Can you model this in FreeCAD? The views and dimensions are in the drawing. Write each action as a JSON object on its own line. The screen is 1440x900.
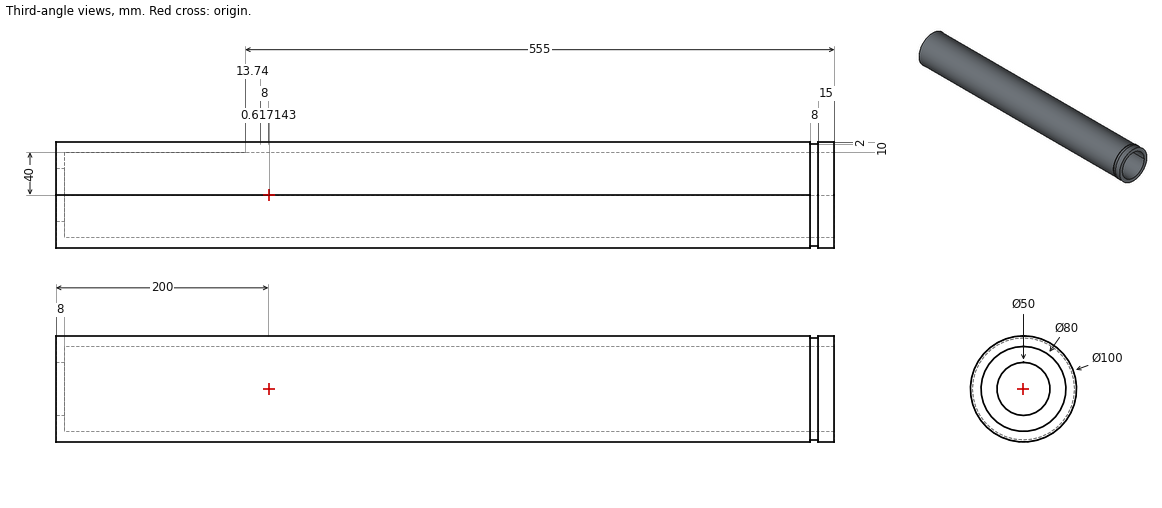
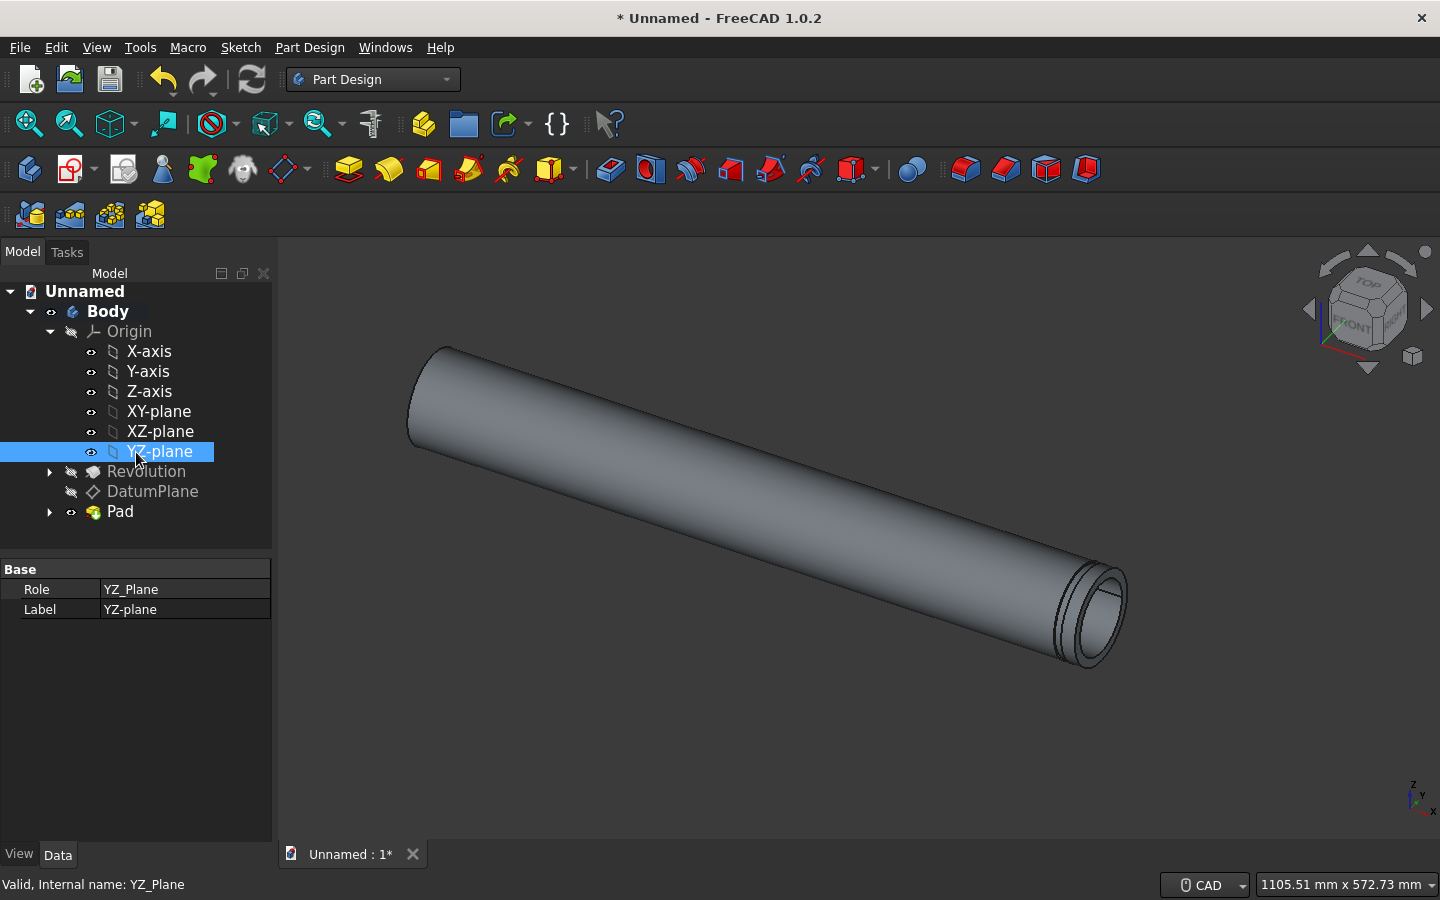
{"action": "left_click", "coordinate": [284, 170]}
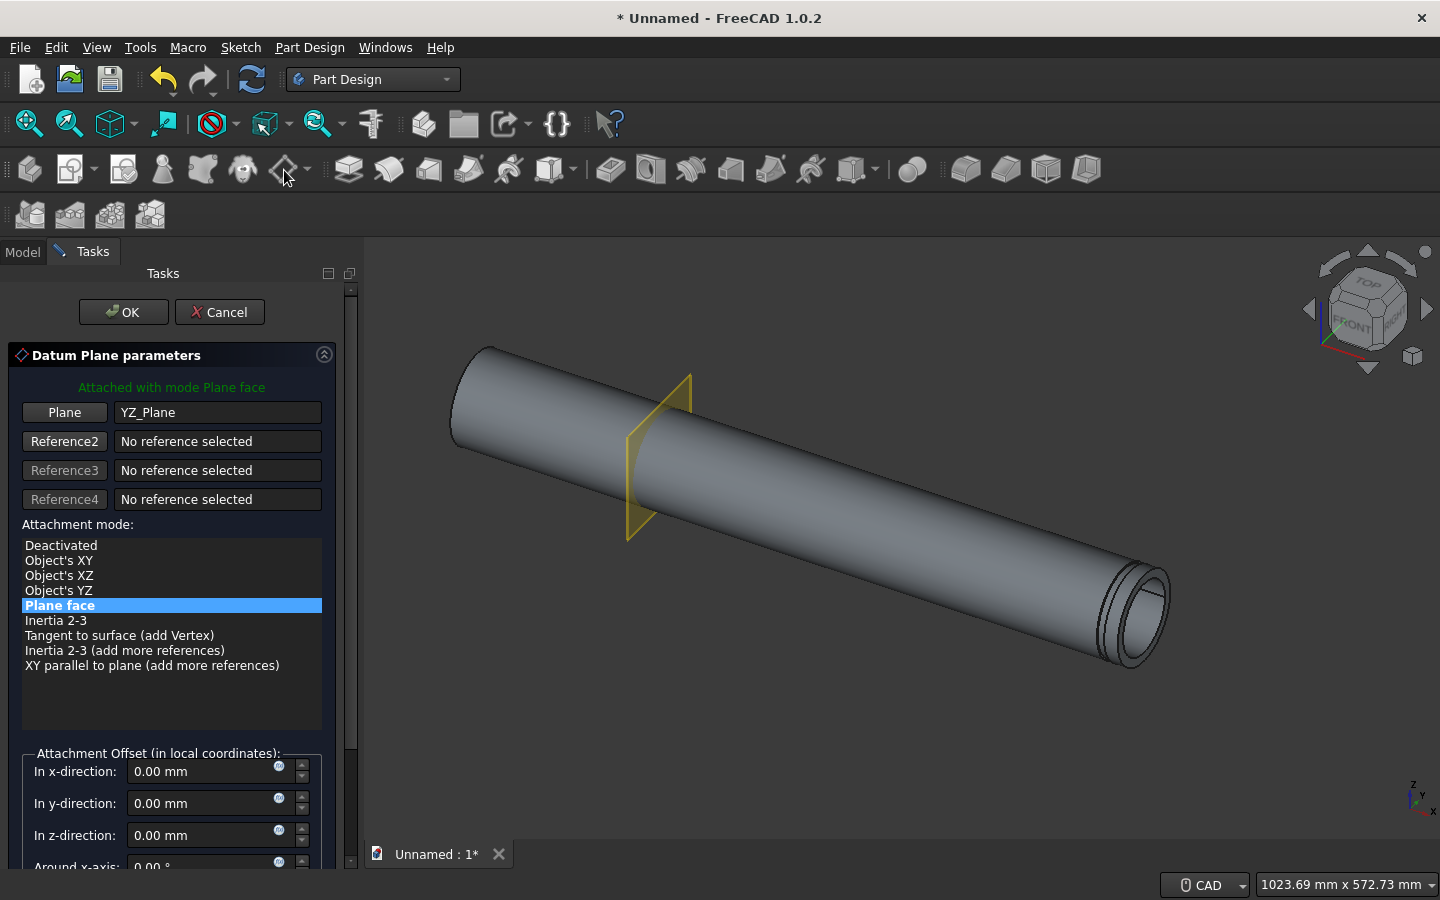
{"action": "triple_click", "coordinate": [210, 835]}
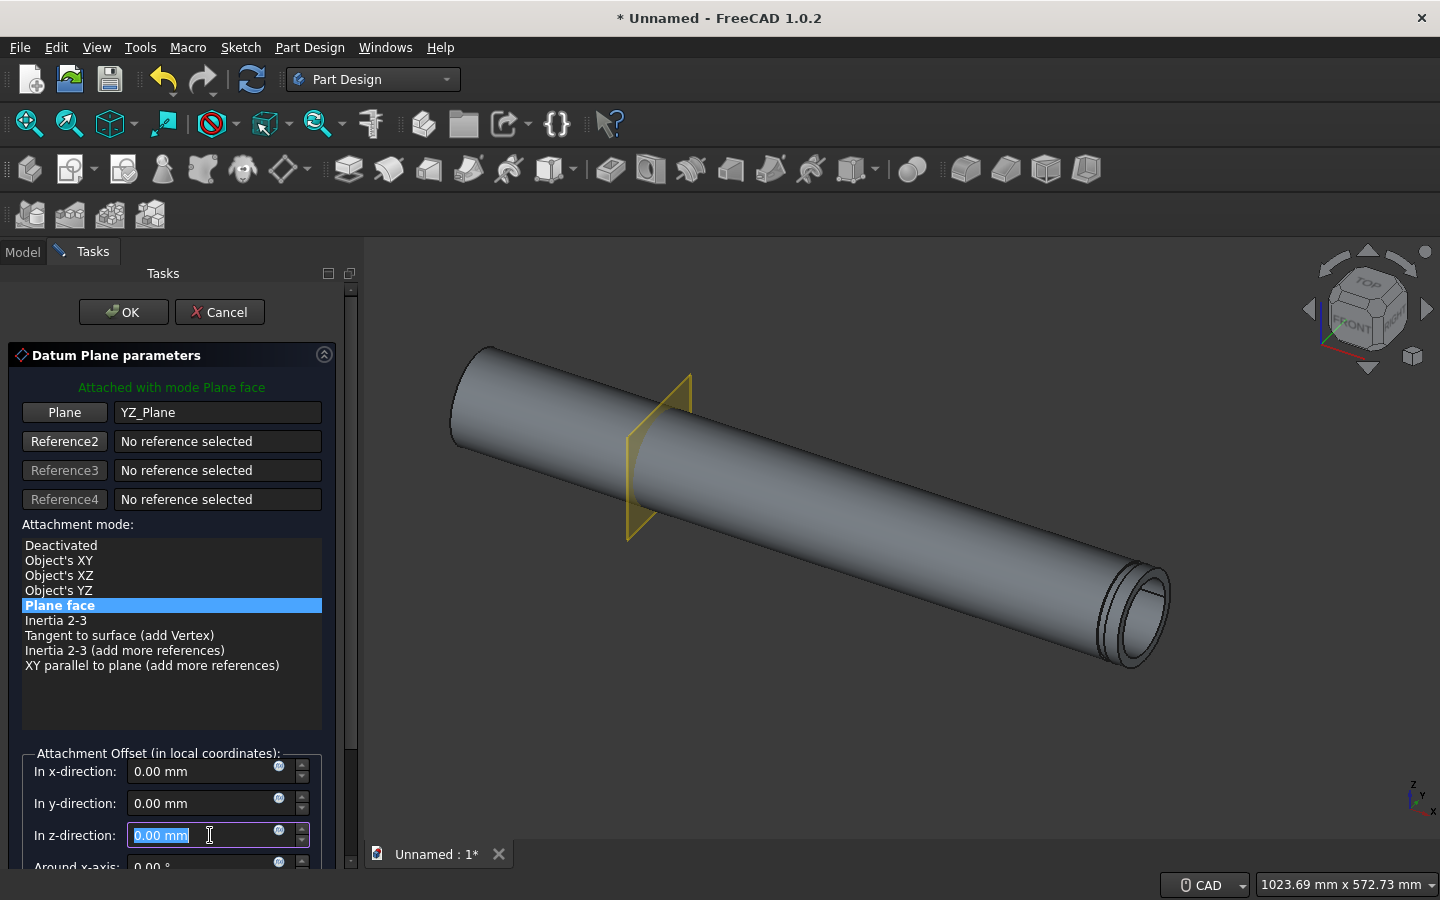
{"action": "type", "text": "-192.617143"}
{"action": "key", "text": "Tab"}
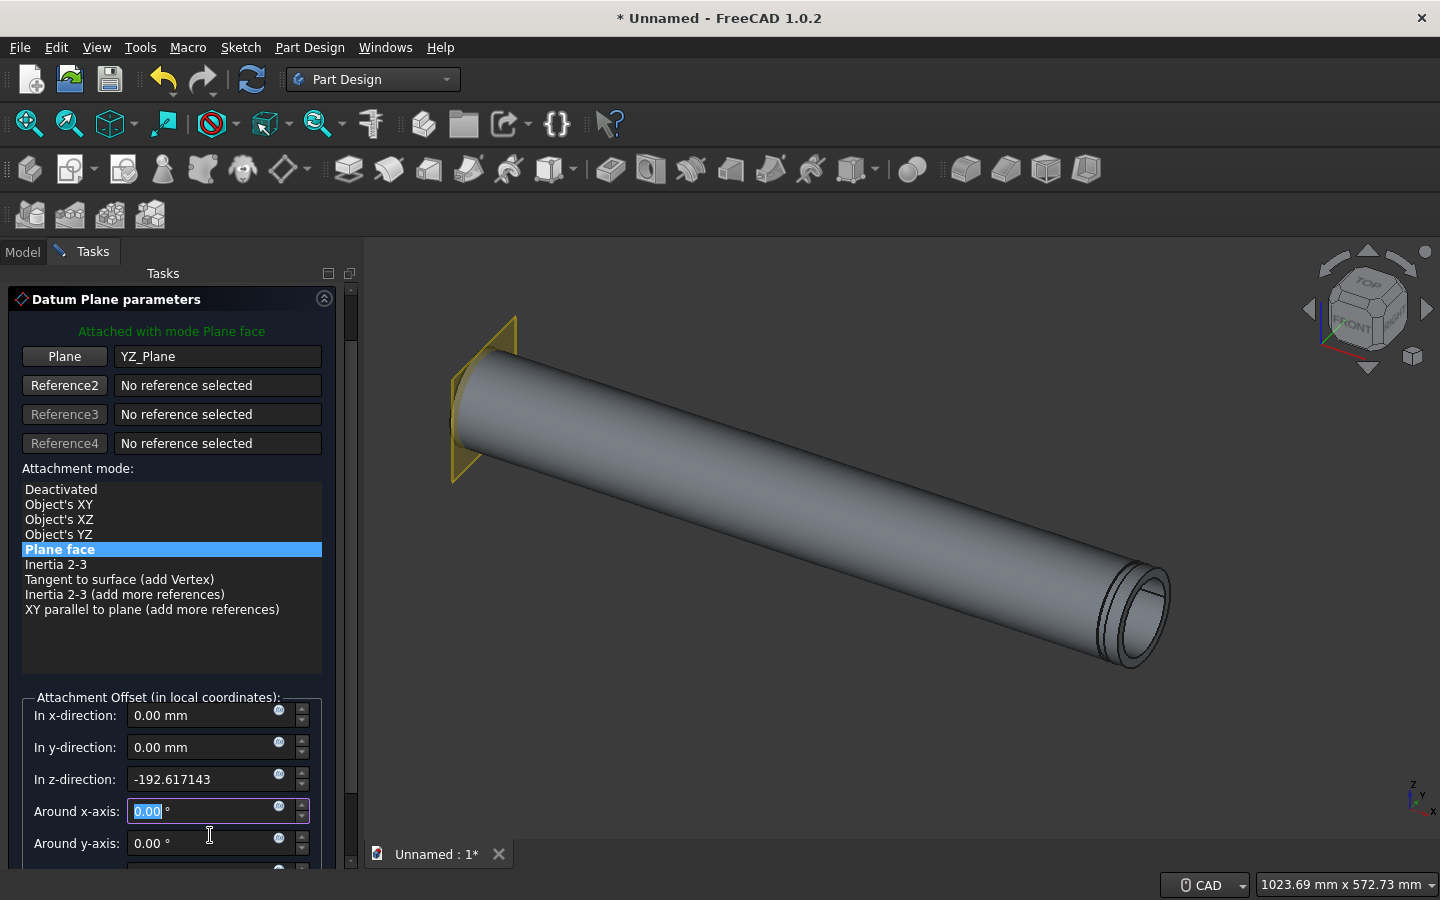
{"action": "scroll", "coordinate": [351, 576], "scroll_direction": "up", "scroll_amount": 2}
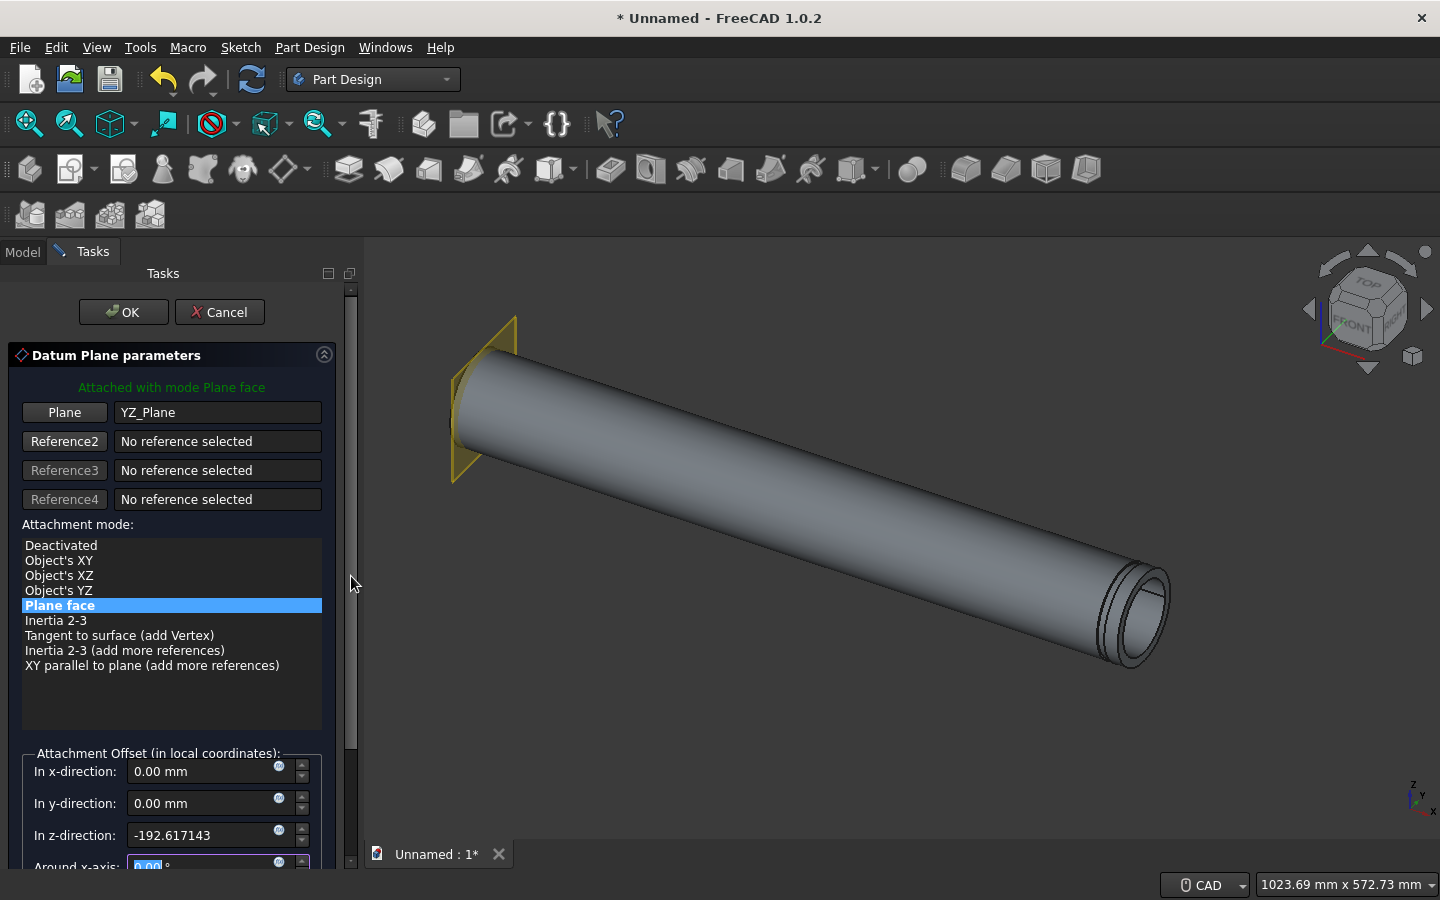
{"action": "left_click", "coordinate": [124, 312]}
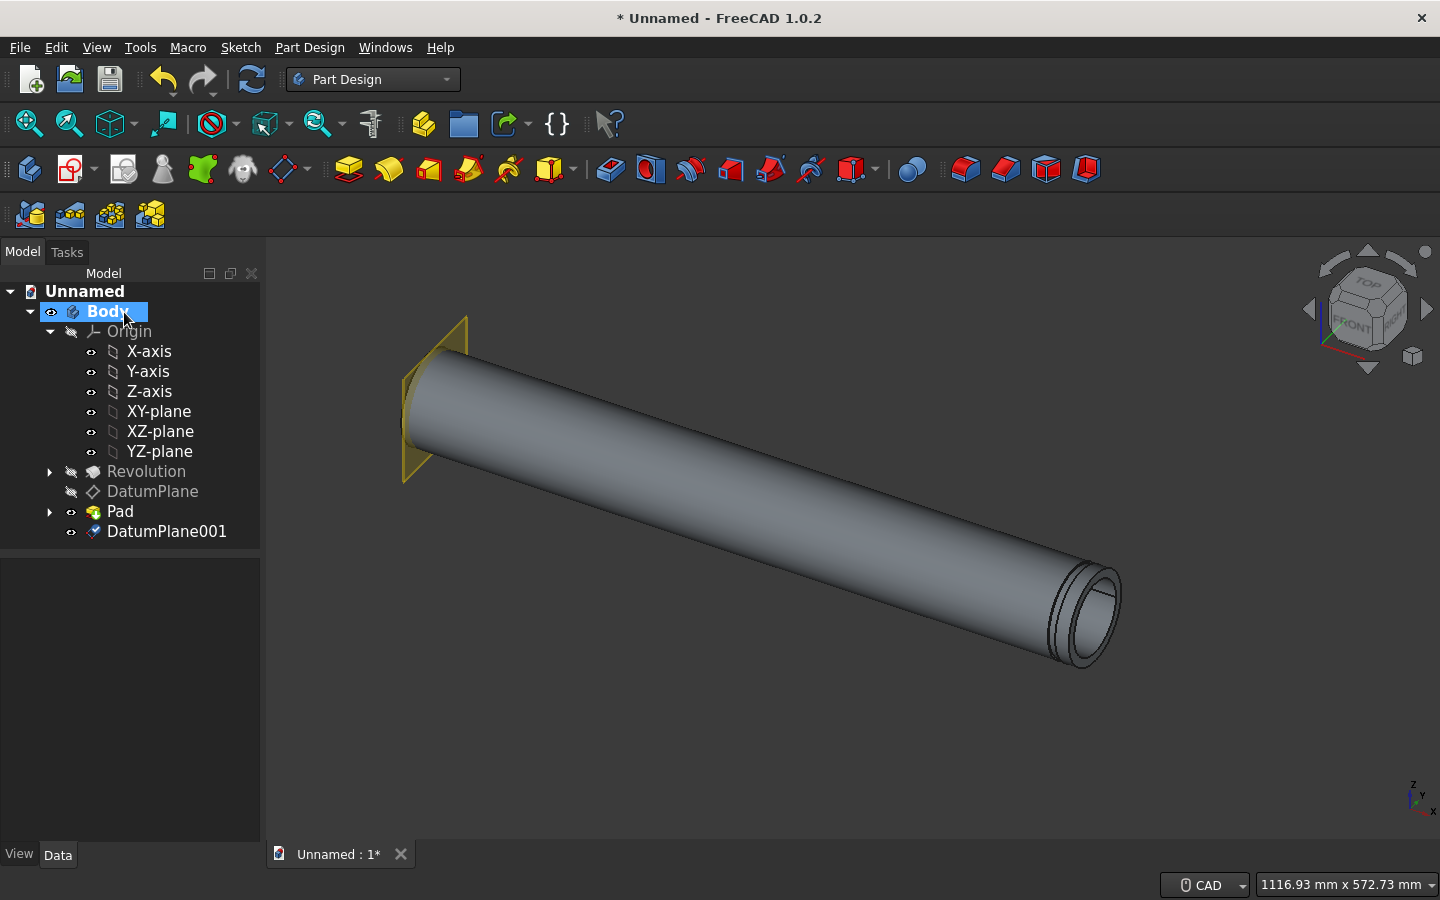
{"action": "left_click", "coordinate": [116, 532]}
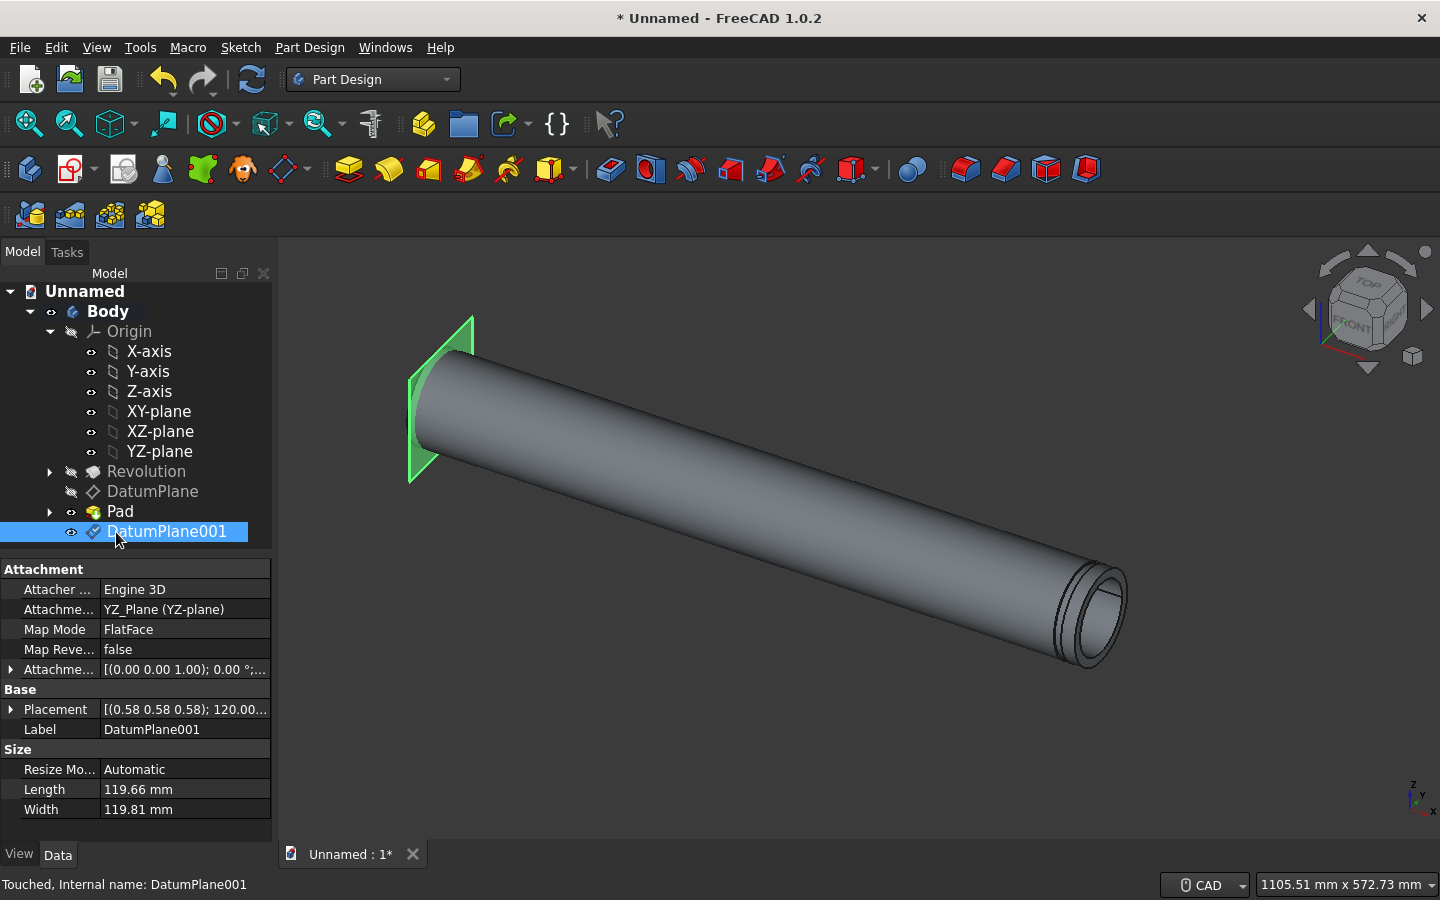
{"action": "left_click", "coordinate": [70, 170]}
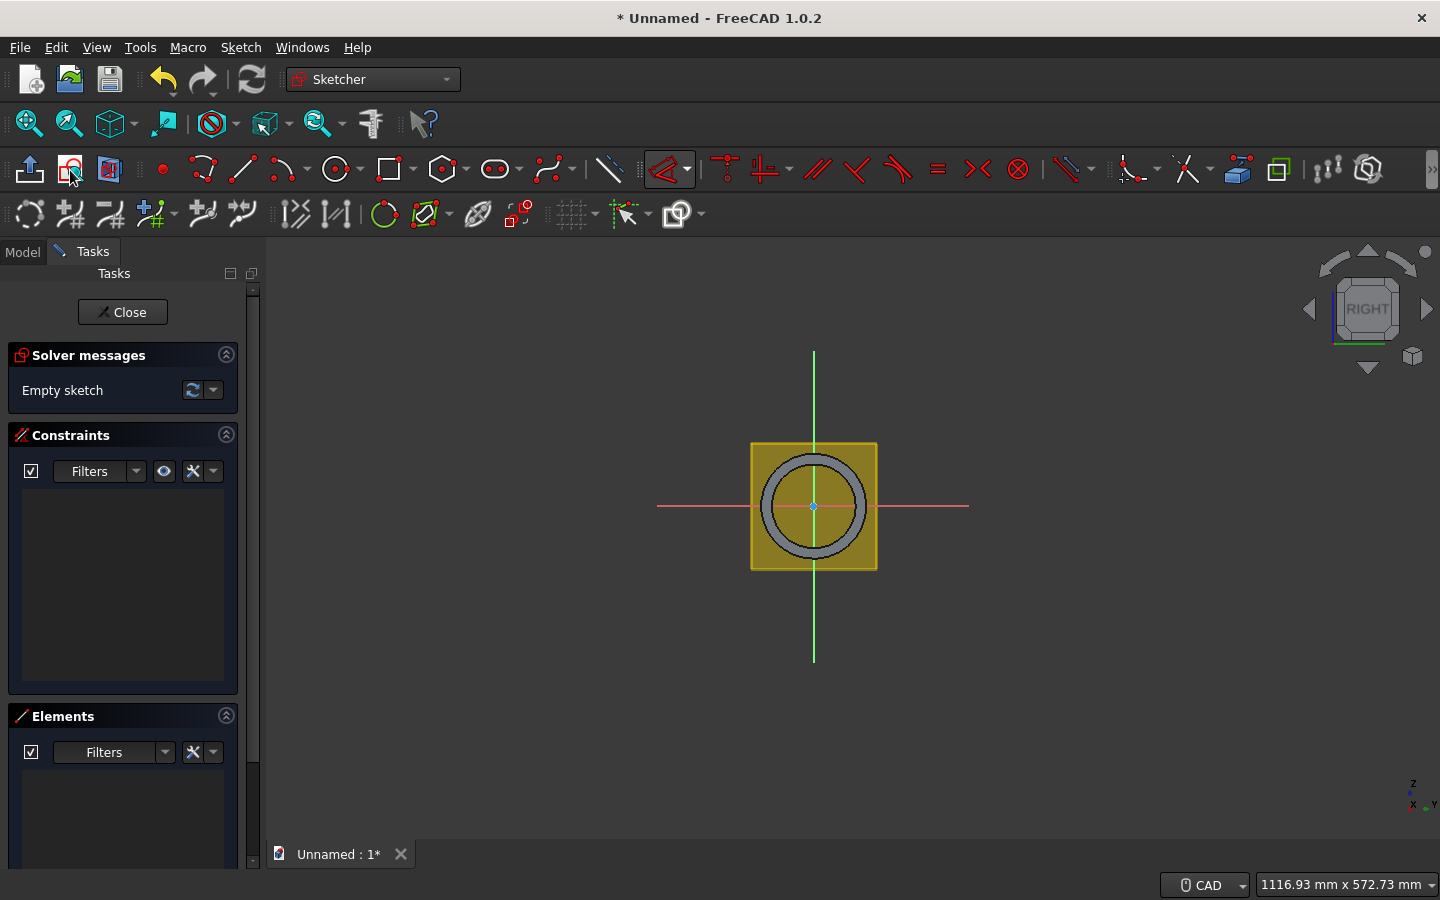
{"action": "left_click", "coordinate": [110, 170]}